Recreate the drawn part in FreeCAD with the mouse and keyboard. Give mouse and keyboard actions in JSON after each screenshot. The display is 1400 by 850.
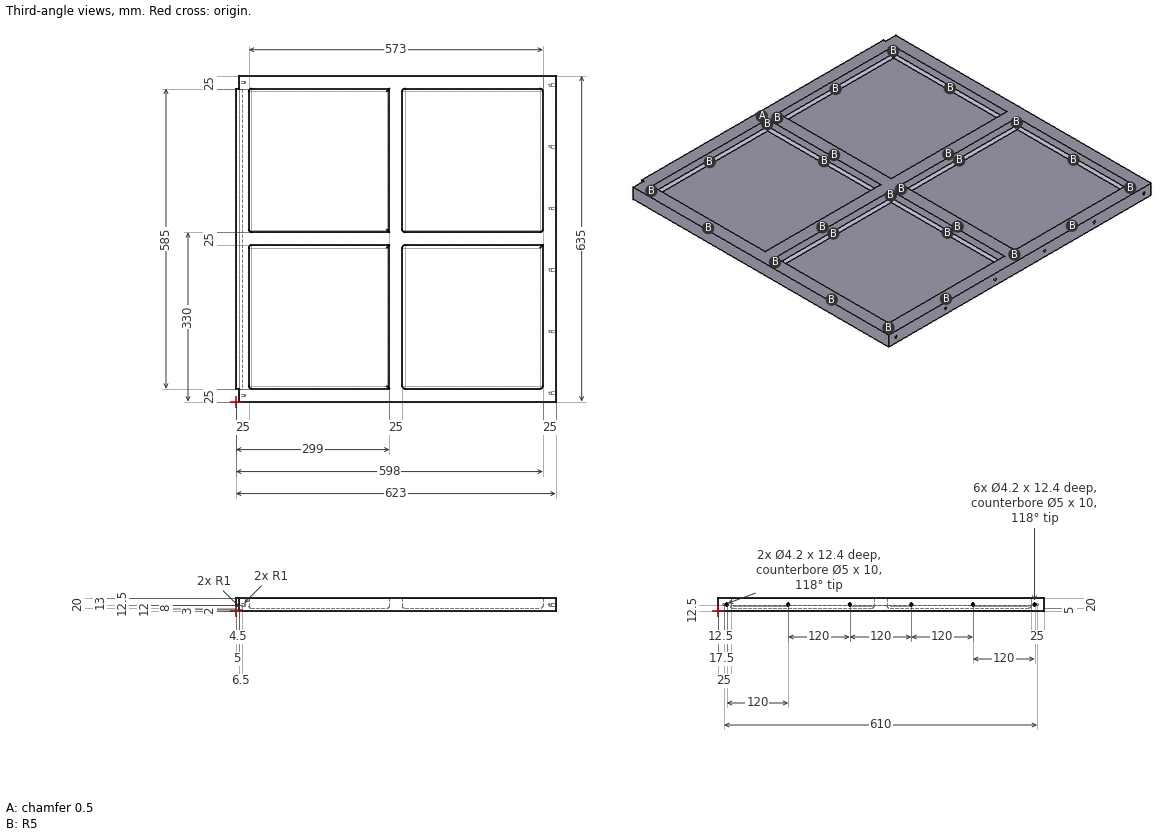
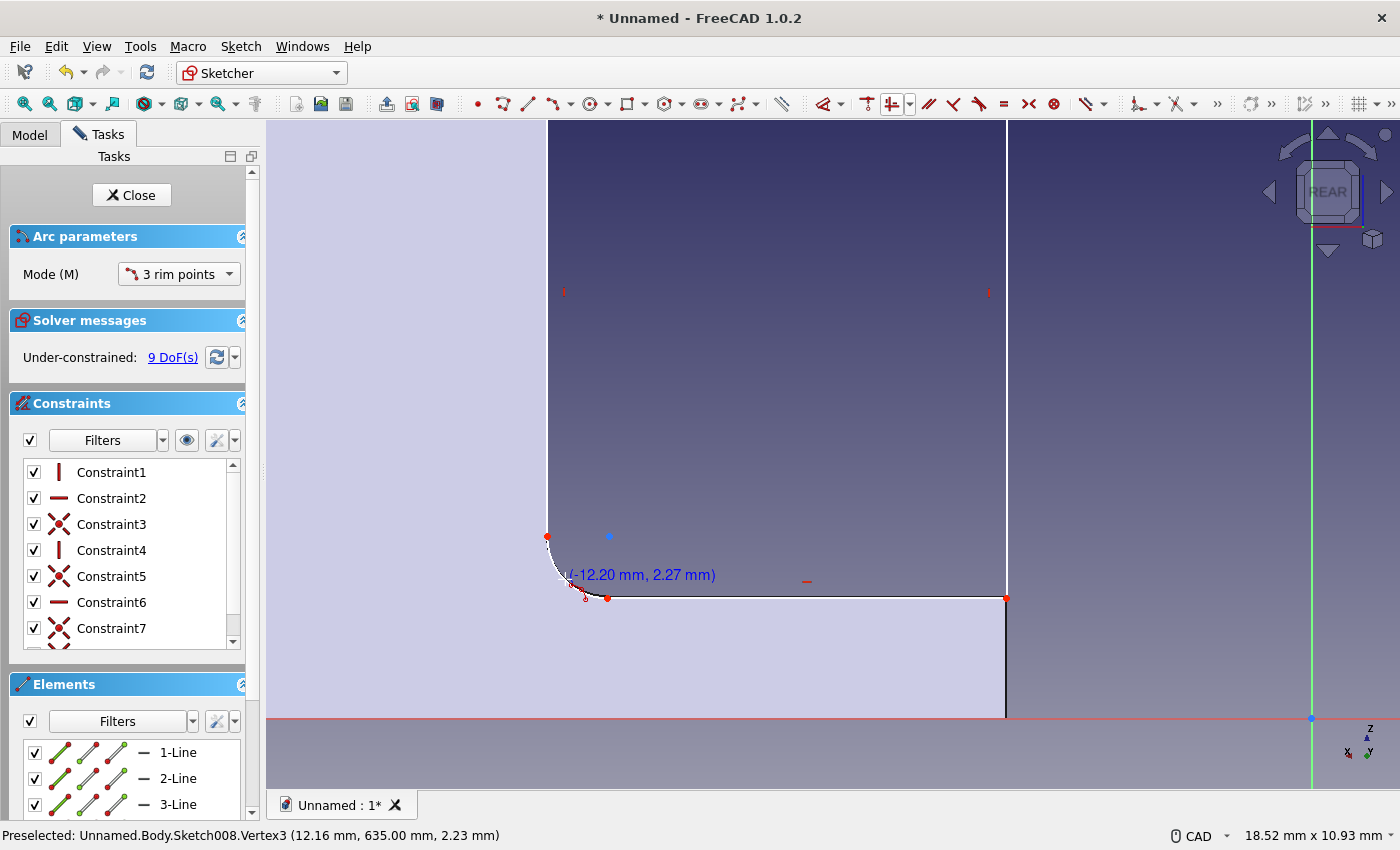
{"action": "scroll", "coordinate": [564, 580], "scroll_direction": "down", "scroll_amount": 3}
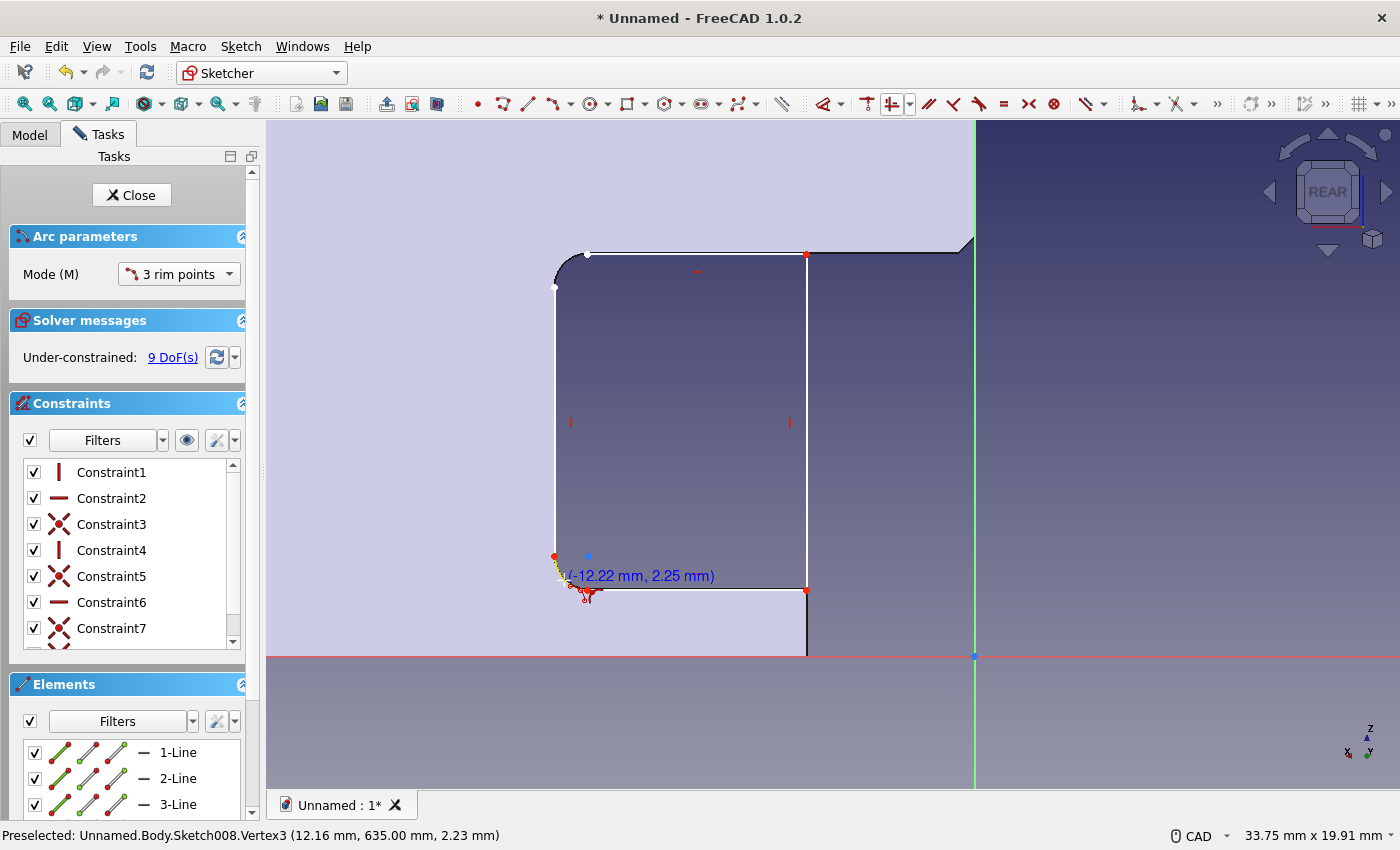
{"action": "left_click", "coordinate": [588, 254]}
{"action": "left_click", "coordinate": [555, 287]}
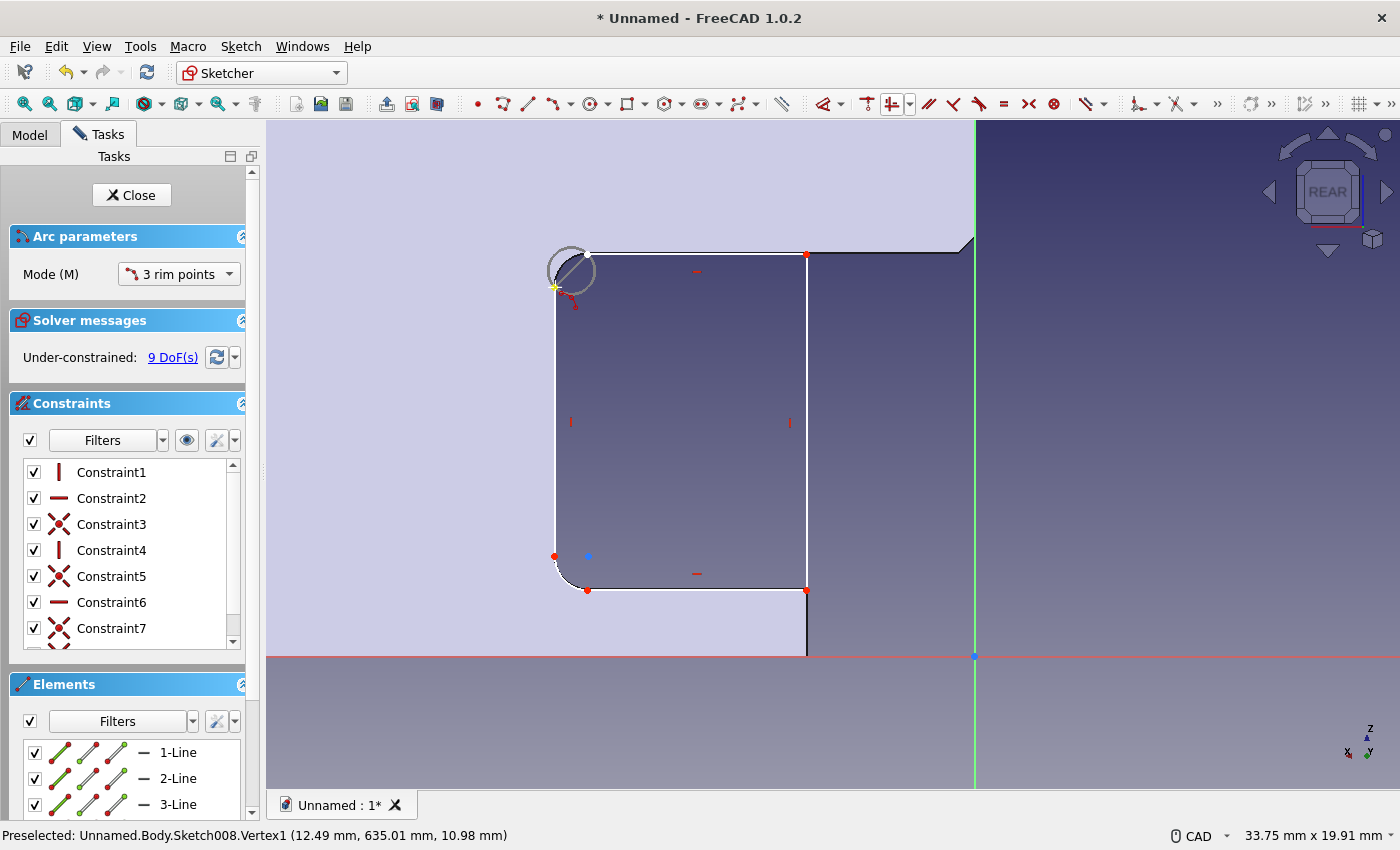
{"action": "scroll", "coordinate": [564, 263], "scroll_direction": "up", "scroll_amount": 3}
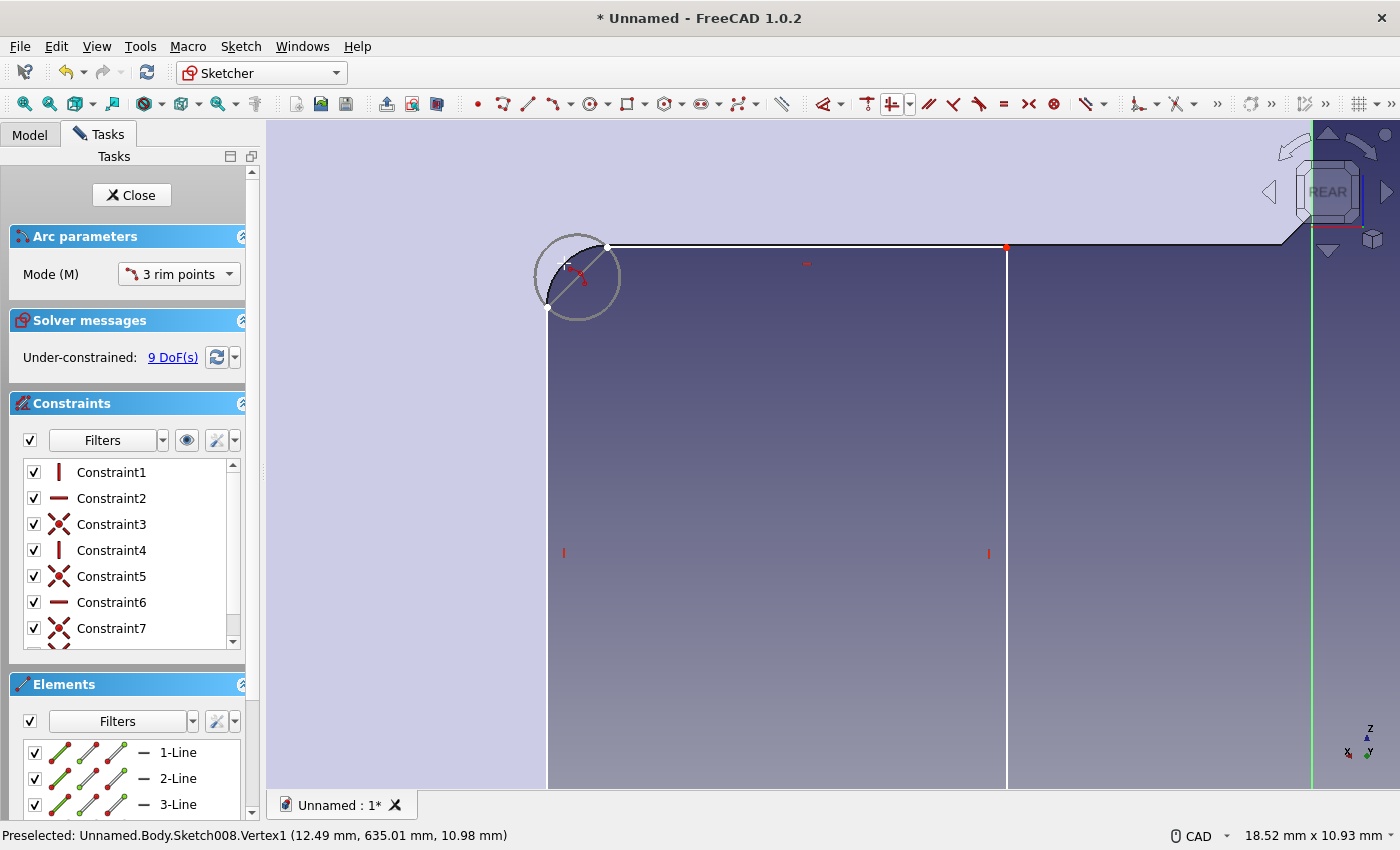
{"action": "left_click", "coordinate": [565, 263]}
{"action": "key", "text": "Escape"}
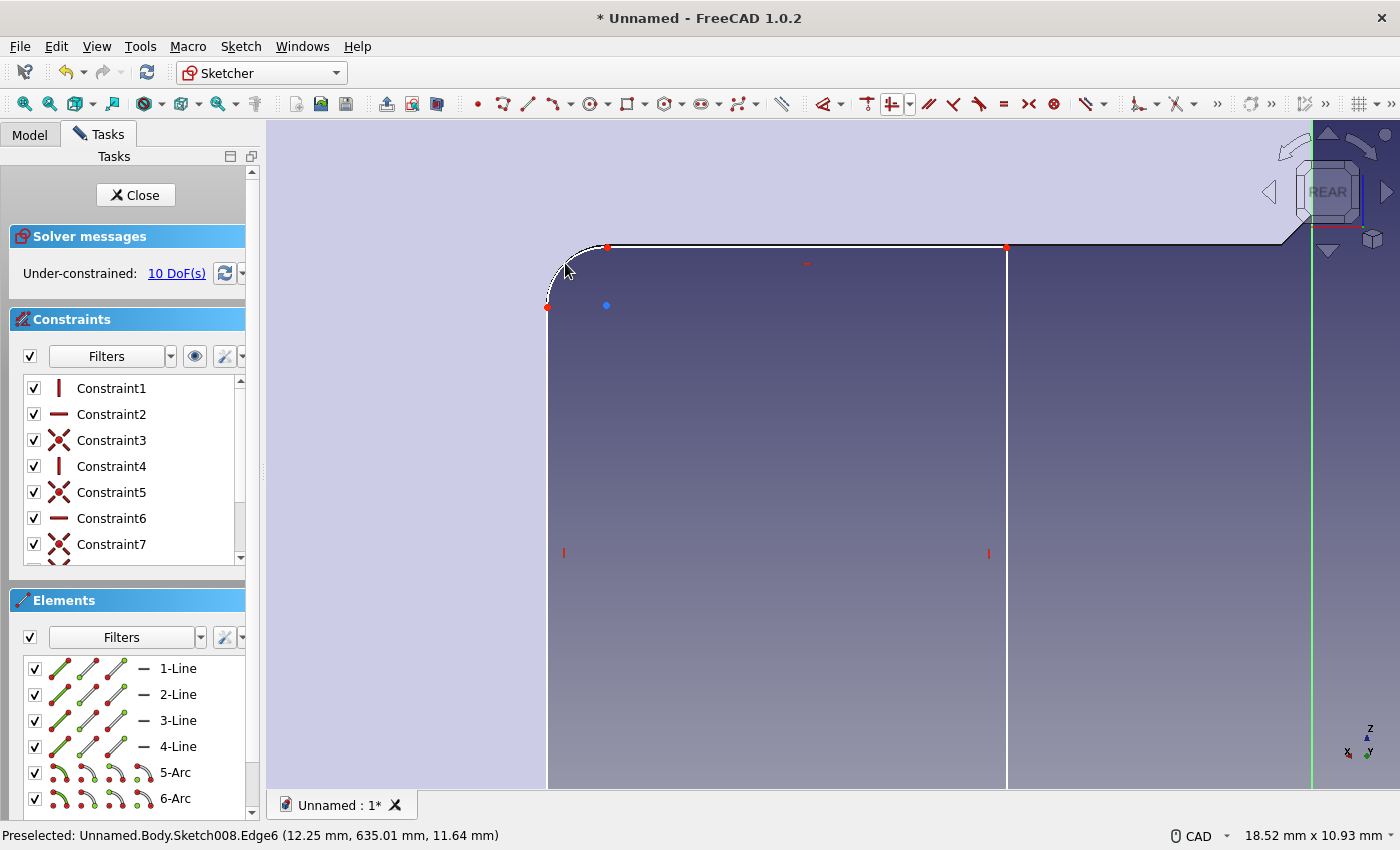
{"action": "left_click", "coordinate": [547, 454]}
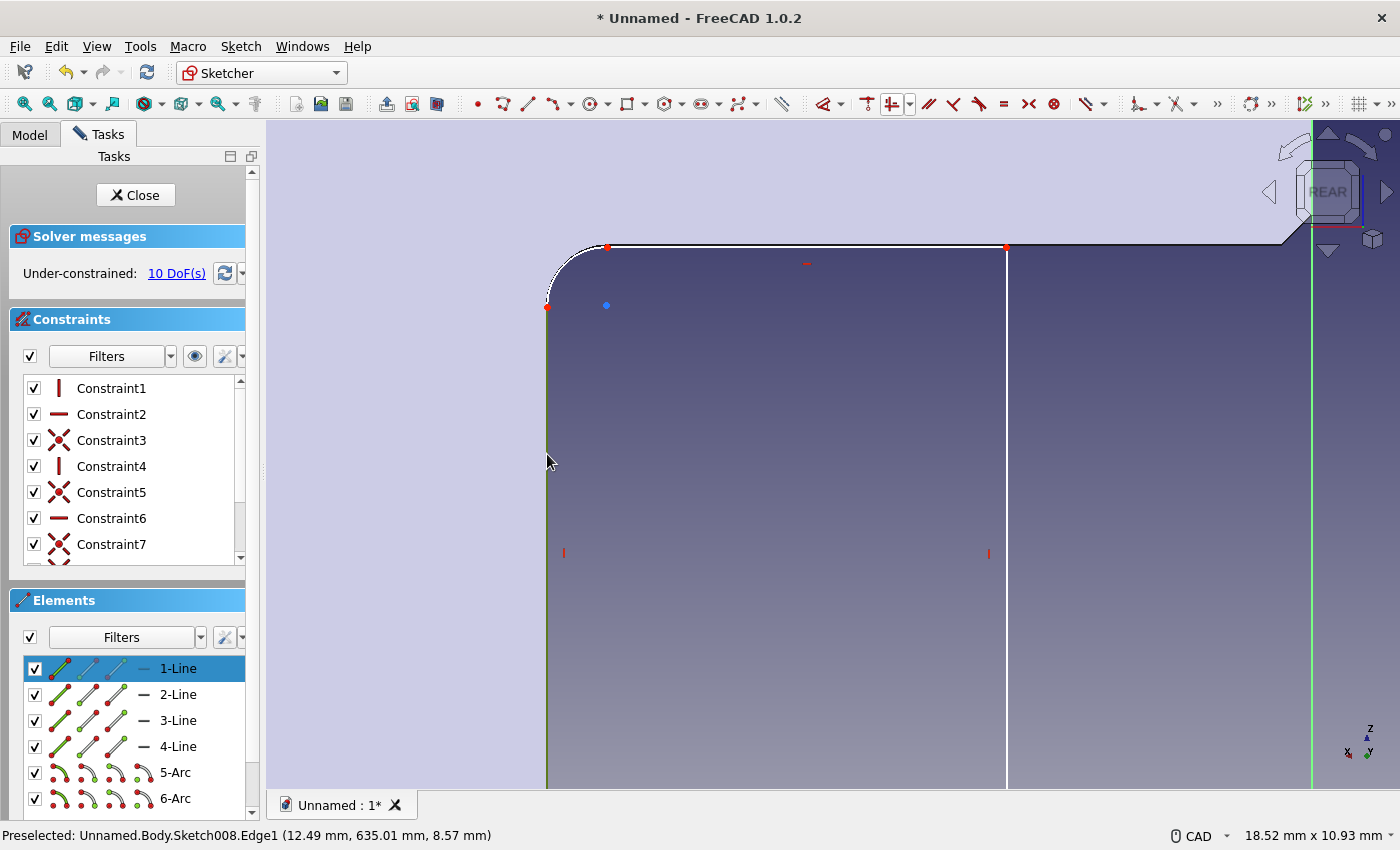
{"action": "scroll", "coordinate": [564, 262], "scroll_direction": "down", "scroll_amount": 3}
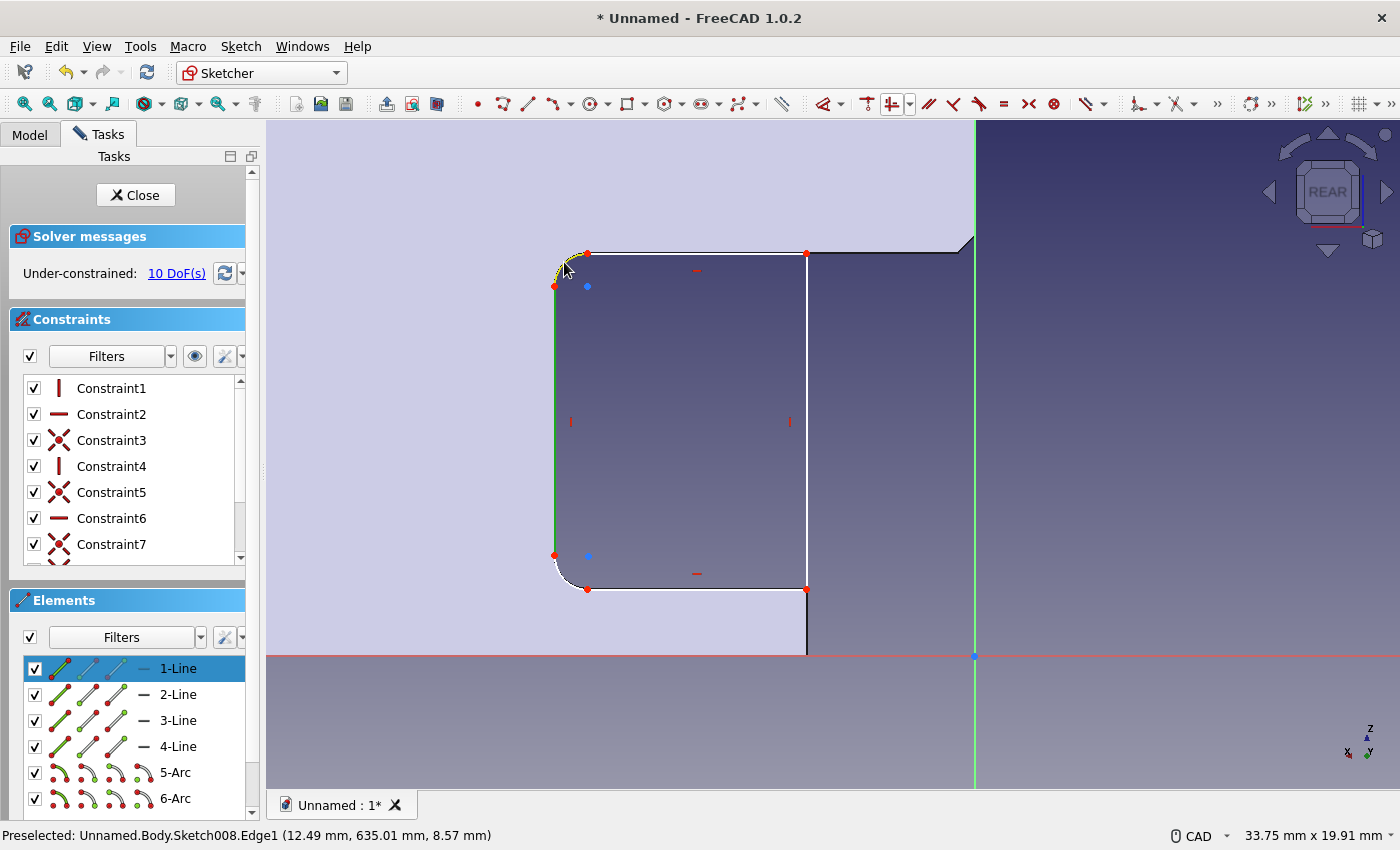
{"action": "left_click", "coordinate": [559, 571]}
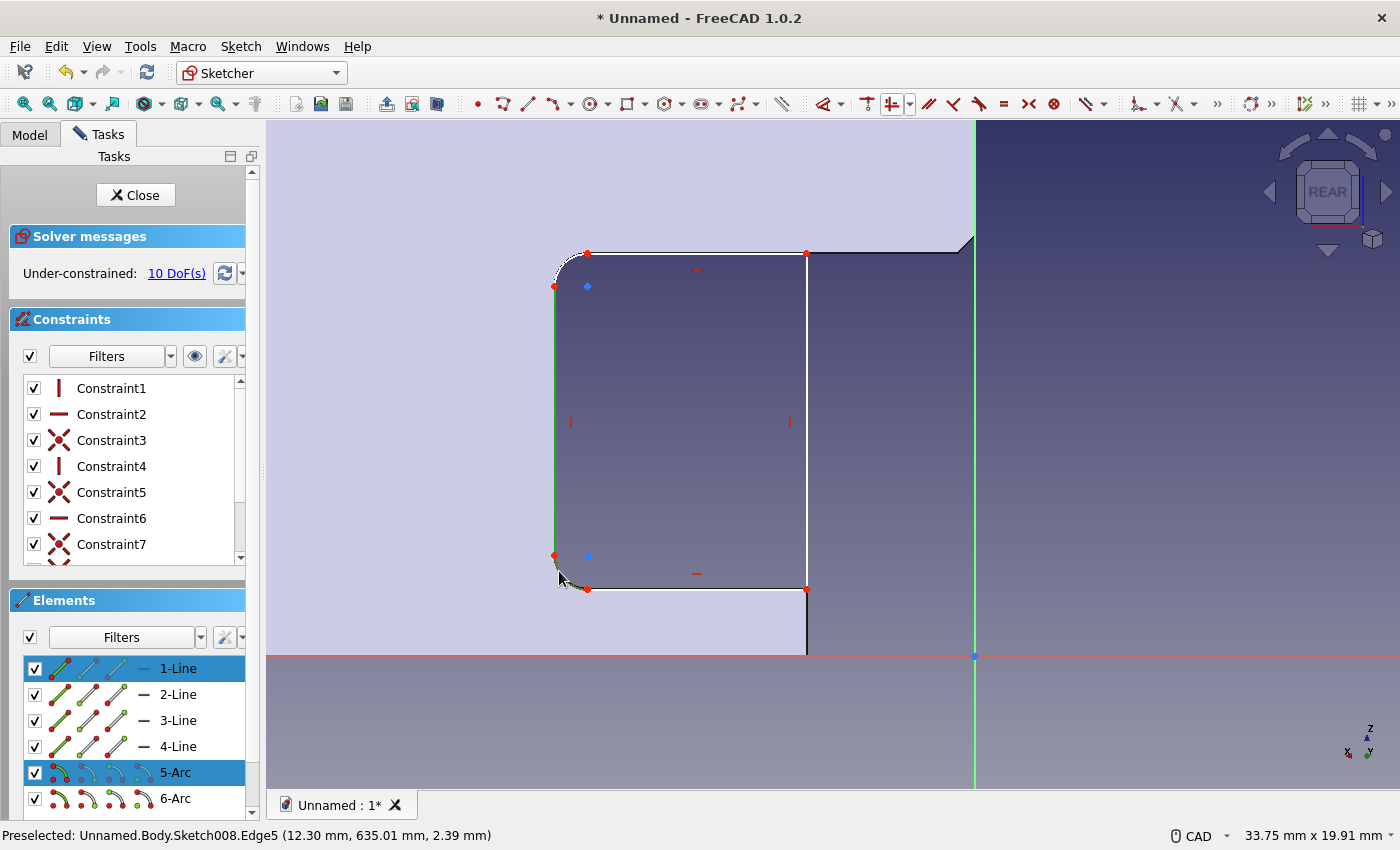
{"action": "left_click", "coordinate": [979, 104]}